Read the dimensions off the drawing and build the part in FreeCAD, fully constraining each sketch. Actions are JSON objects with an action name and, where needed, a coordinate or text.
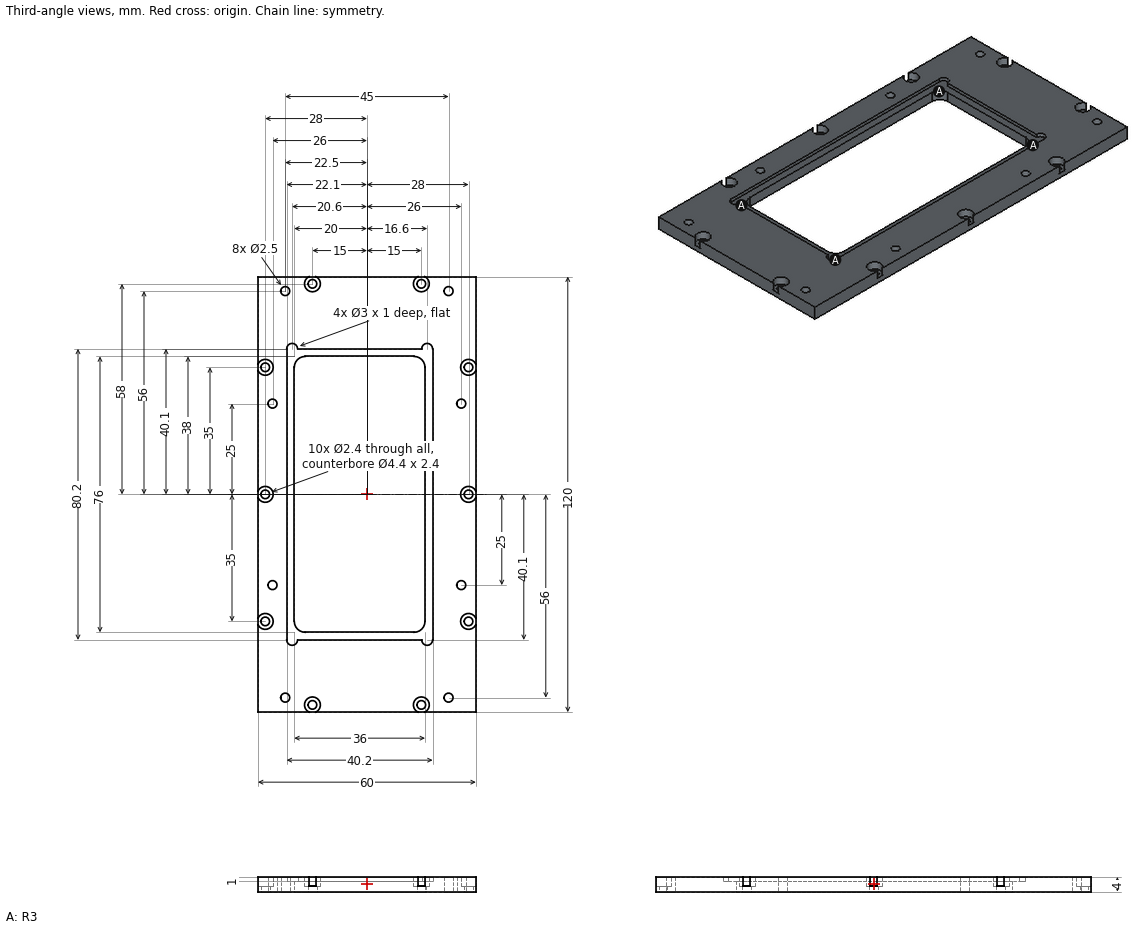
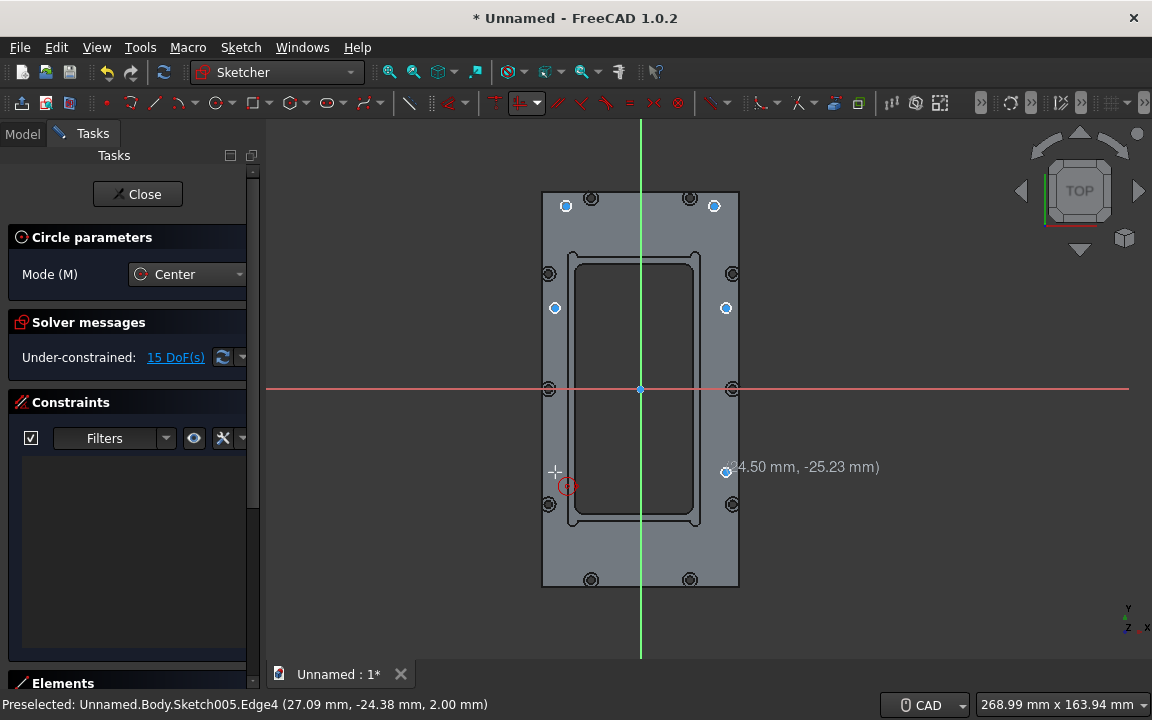
{"action": "left_click", "coordinate": [555, 472]}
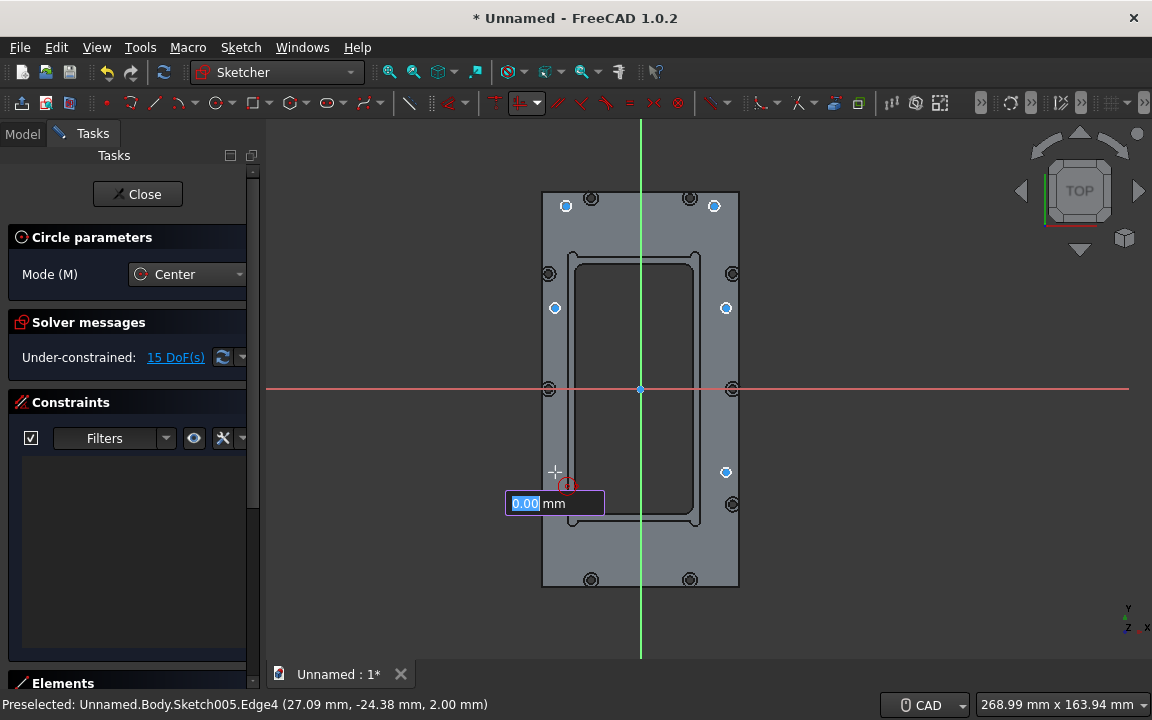
{"action": "scroll", "coordinate": [558, 469], "scroll_direction": "up", "scroll_amount": 7}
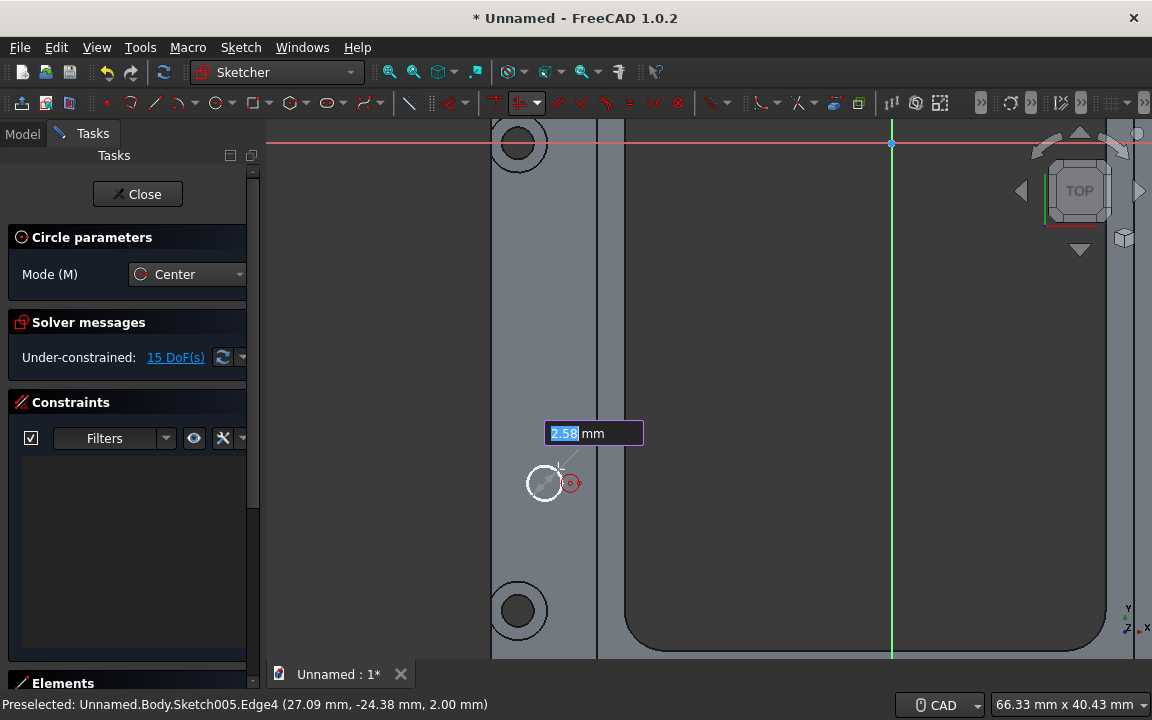
{"action": "left_click", "coordinate": [556, 465]}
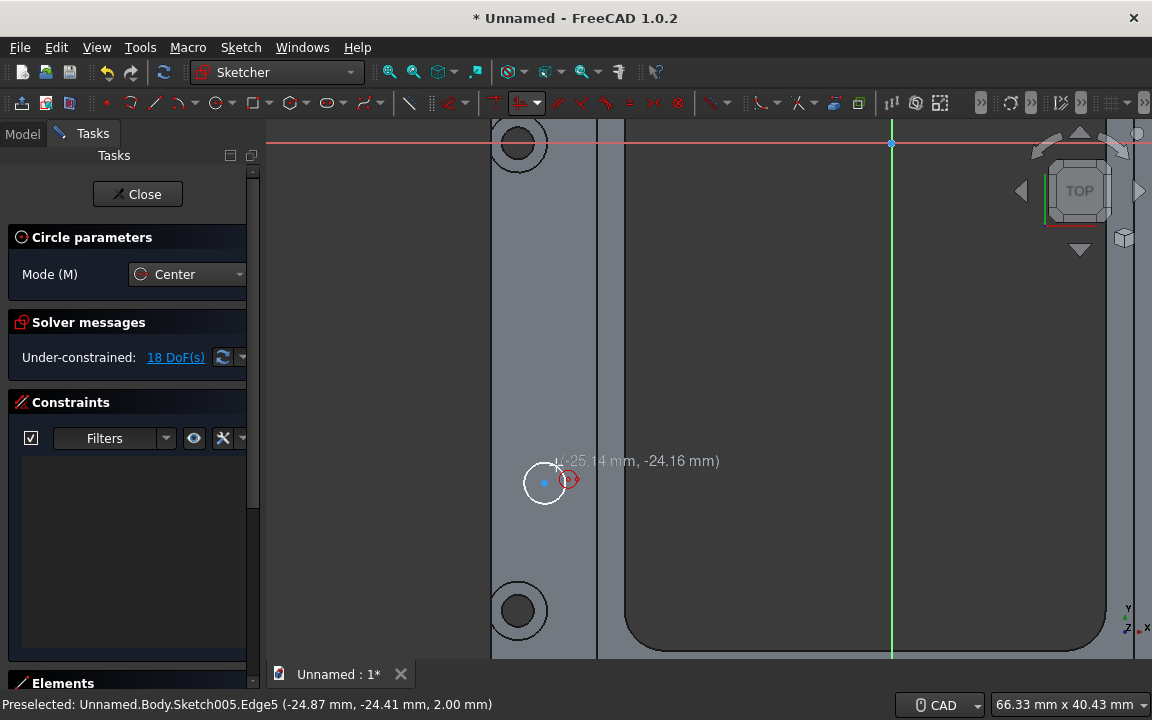
{"action": "scroll", "coordinate": [558, 469], "scroll_direction": "down", "scroll_amount": 7}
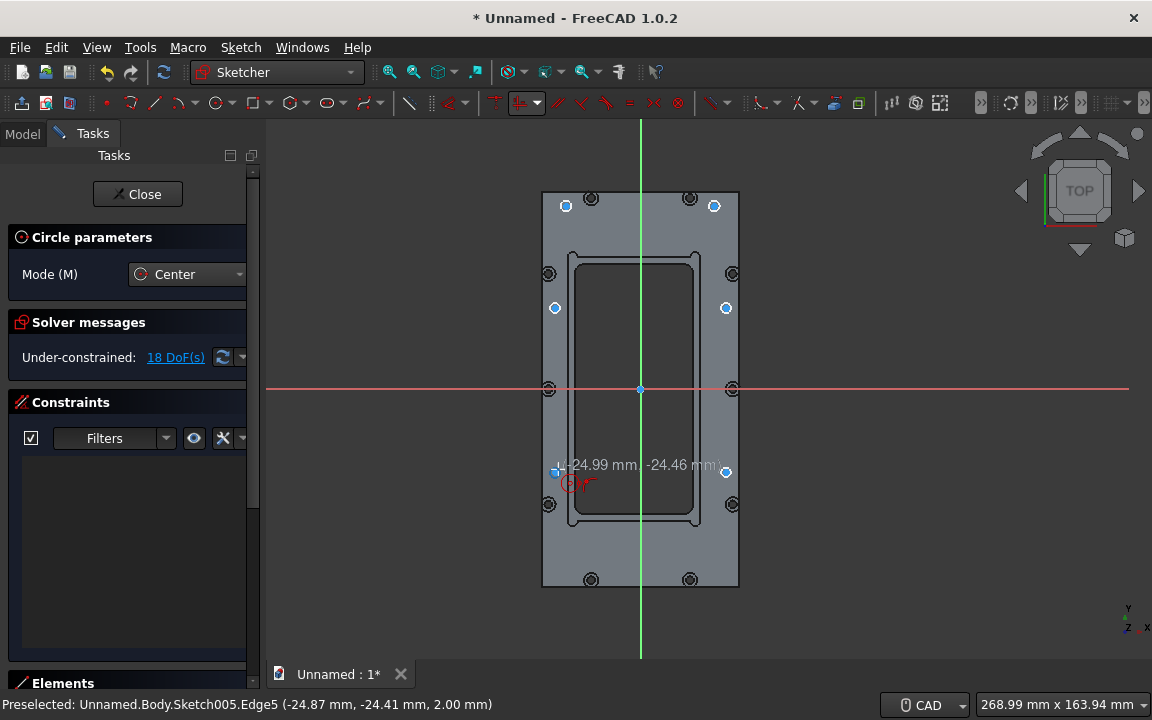
{"action": "scroll", "coordinate": [715, 574], "scroll_direction": "up", "scroll_amount": 9}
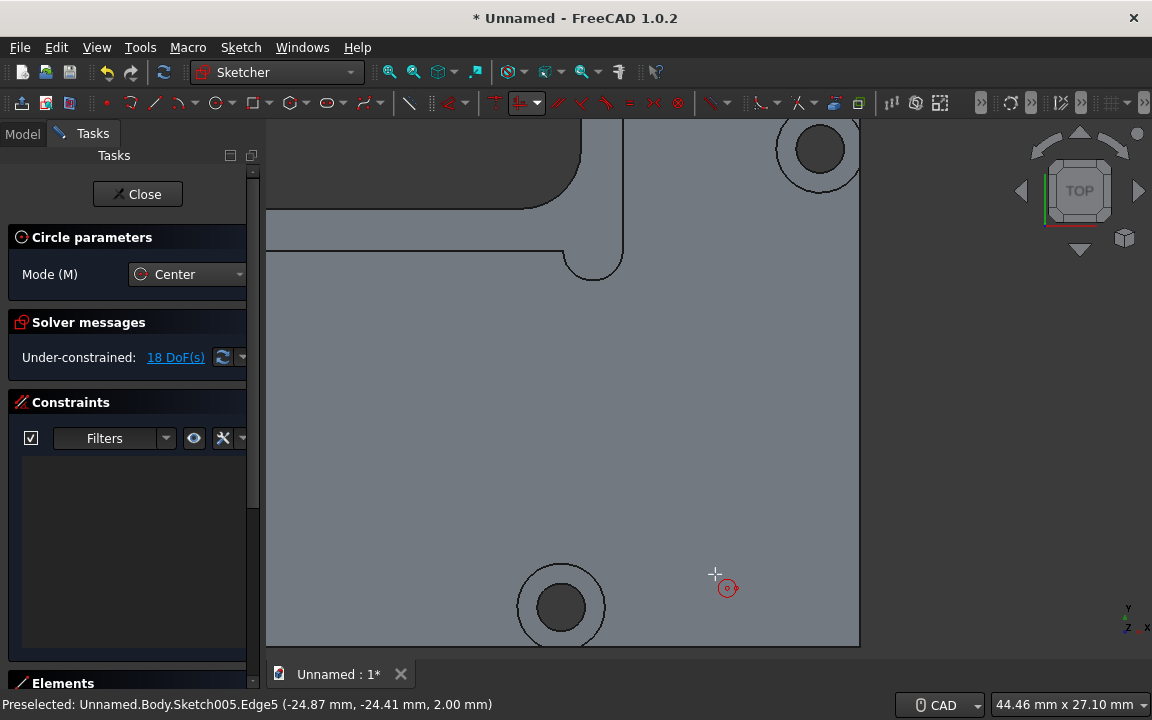
{"action": "scroll", "coordinate": [715, 575], "scroll_direction": "down", "scroll_amount": 9}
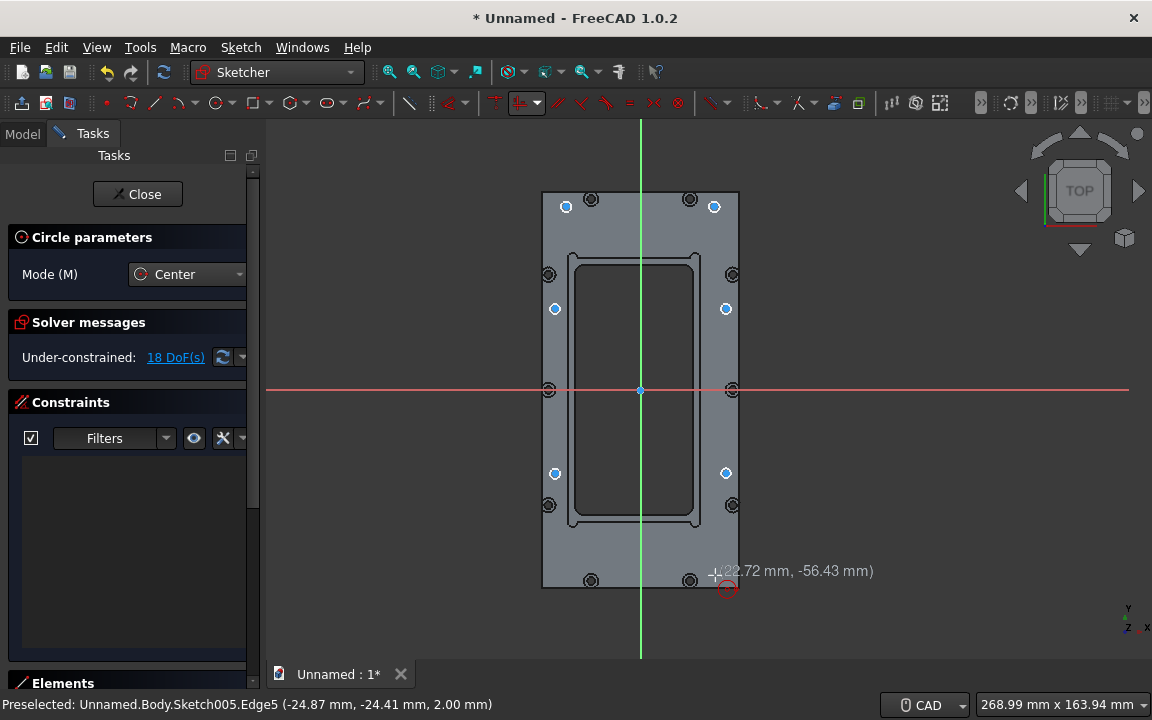
{"action": "left_click", "coordinate": [715, 574]}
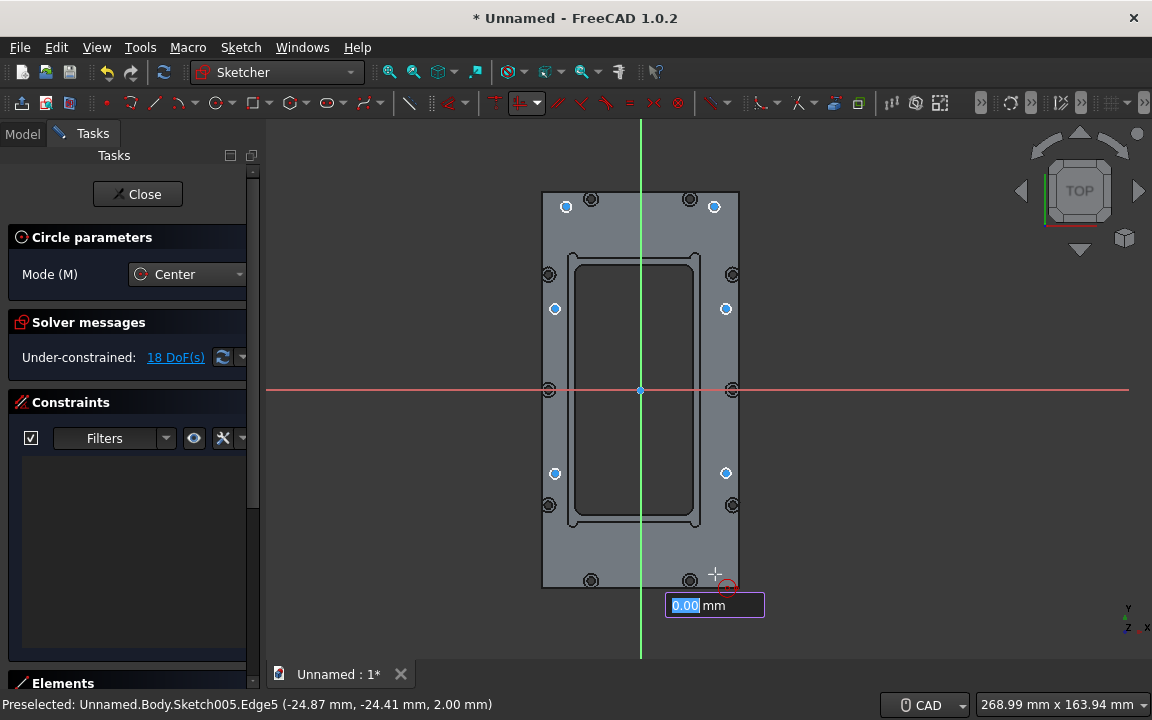
{"action": "scroll", "coordinate": [718, 572], "scroll_direction": "up", "scroll_amount": 7}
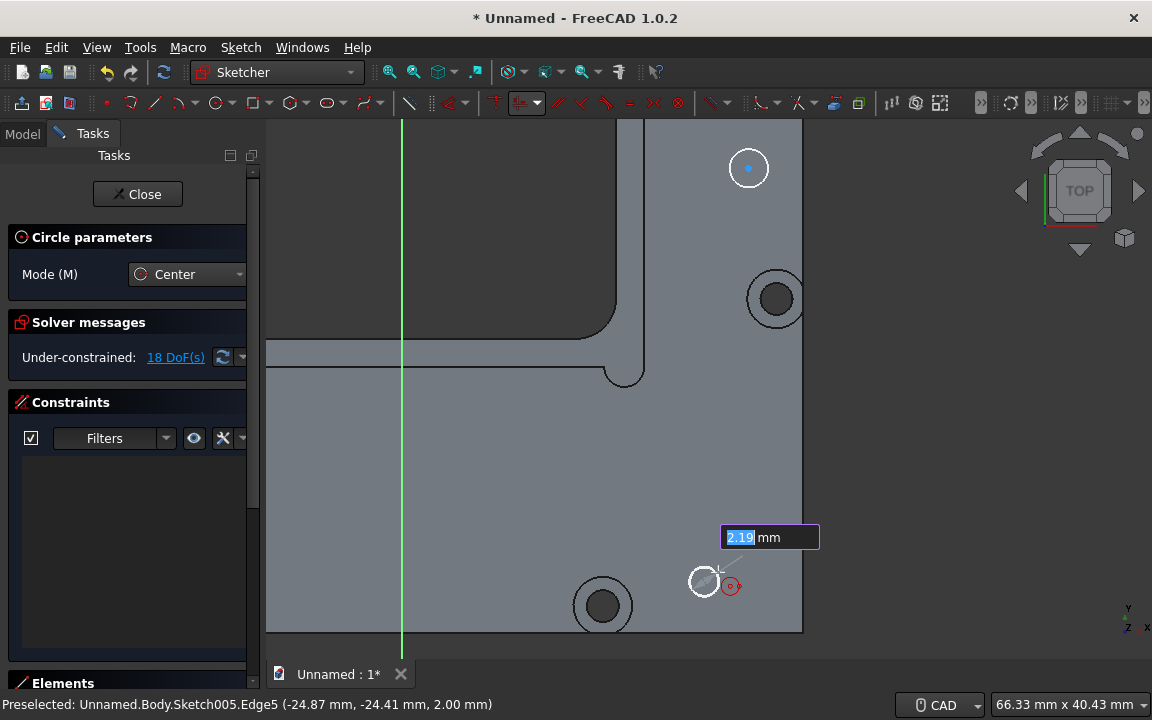
{"action": "left_click", "coordinate": [715, 568]}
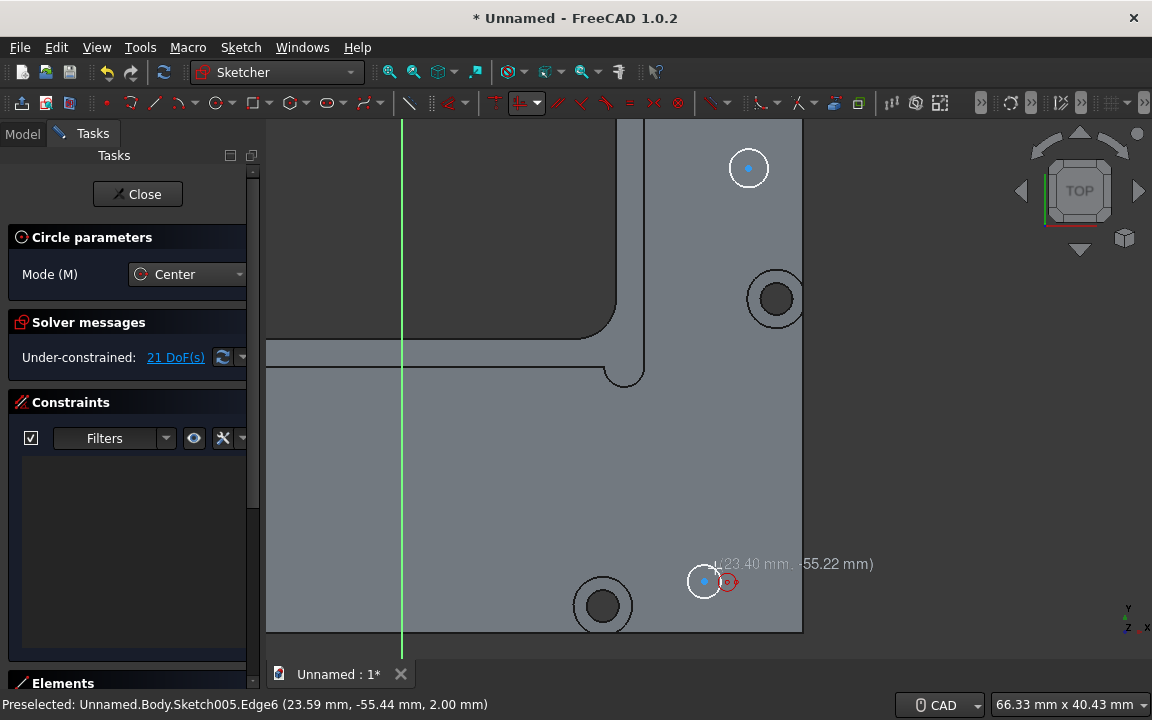
{"action": "scroll", "coordinate": [718, 572], "scroll_direction": "down", "scroll_amount": 7}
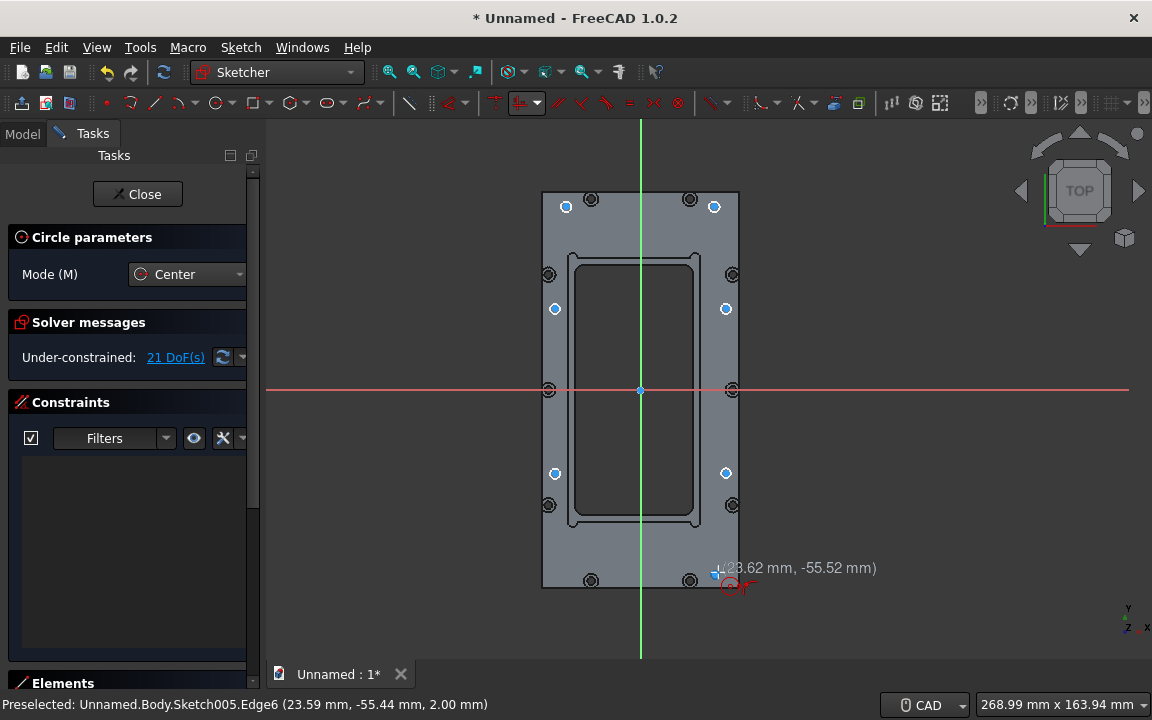
{"action": "scroll", "coordinate": [566, 574], "scroll_direction": "up", "scroll_amount": 9}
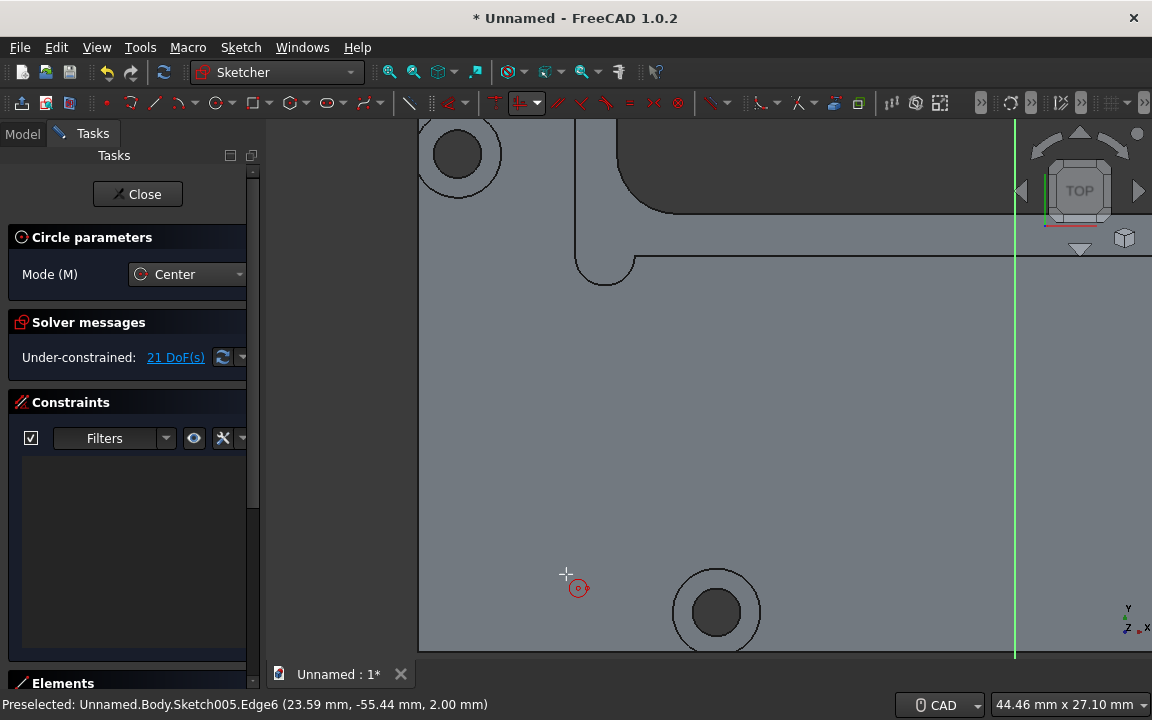
{"action": "scroll", "coordinate": [566, 574], "scroll_direction": "down", "scroll_amount": 9}